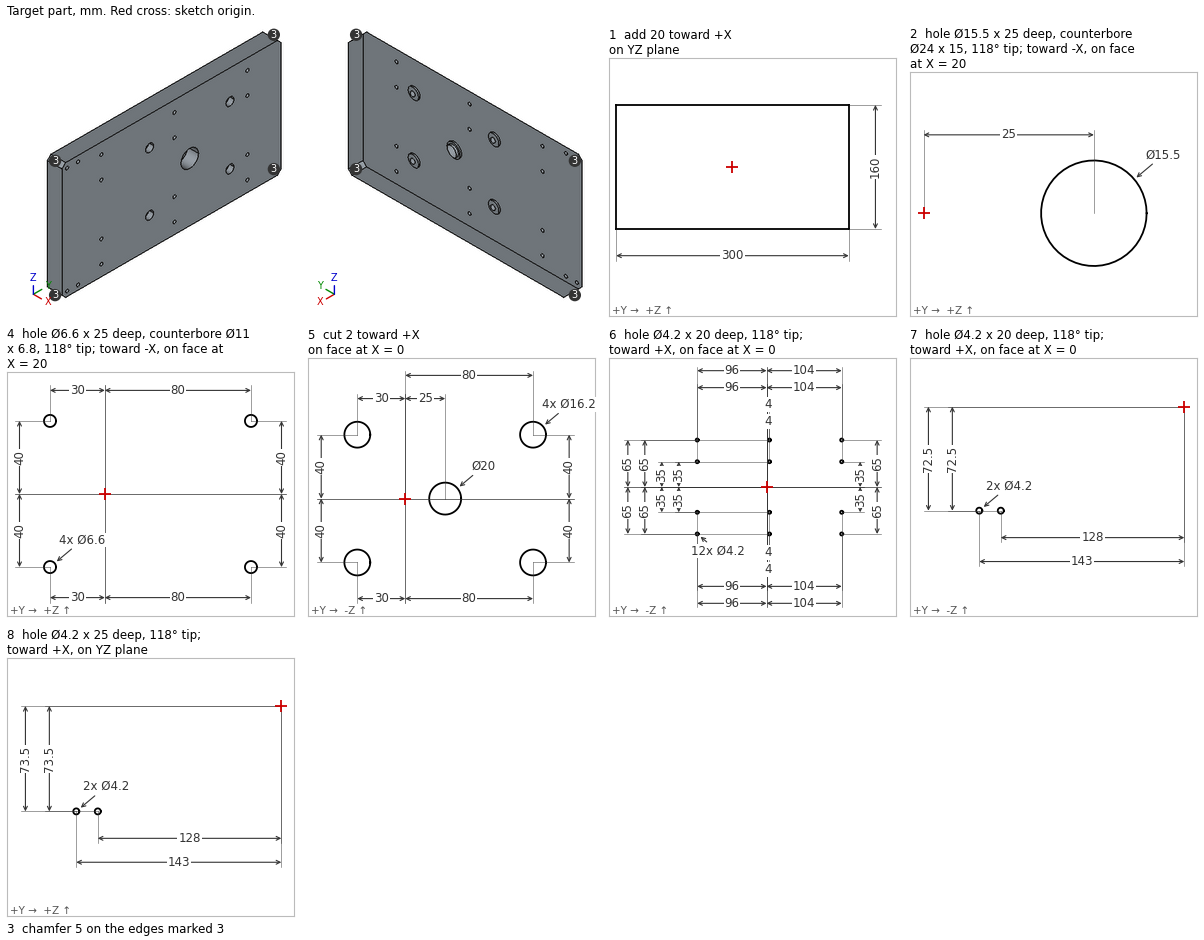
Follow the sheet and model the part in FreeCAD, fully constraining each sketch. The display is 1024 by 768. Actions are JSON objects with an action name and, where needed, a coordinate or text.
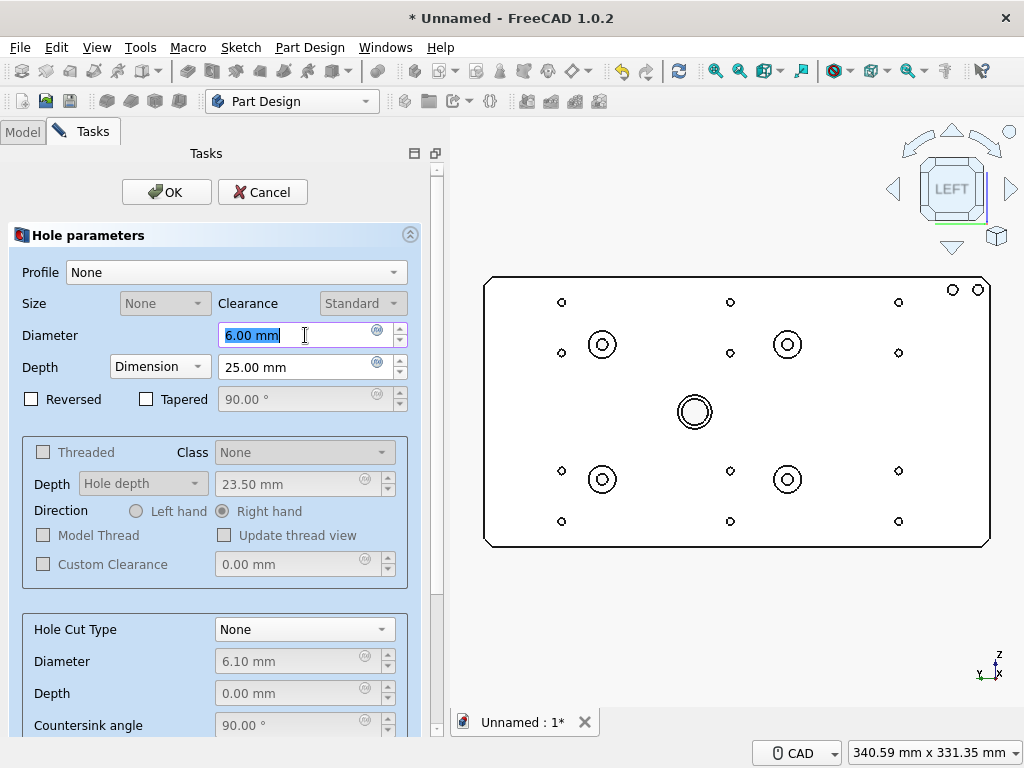
{"action": "type", "text": "4.2"}
{"action": "key", "text": "Tab"}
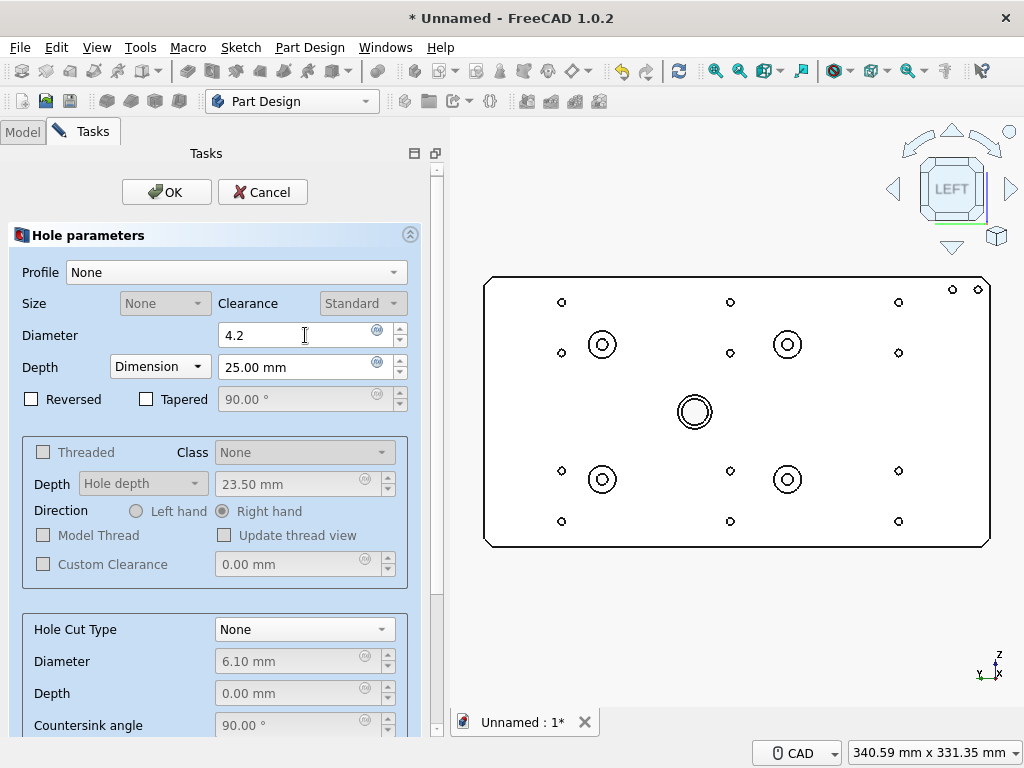
{"action": "triple_click", "coordinate": [305, 367]}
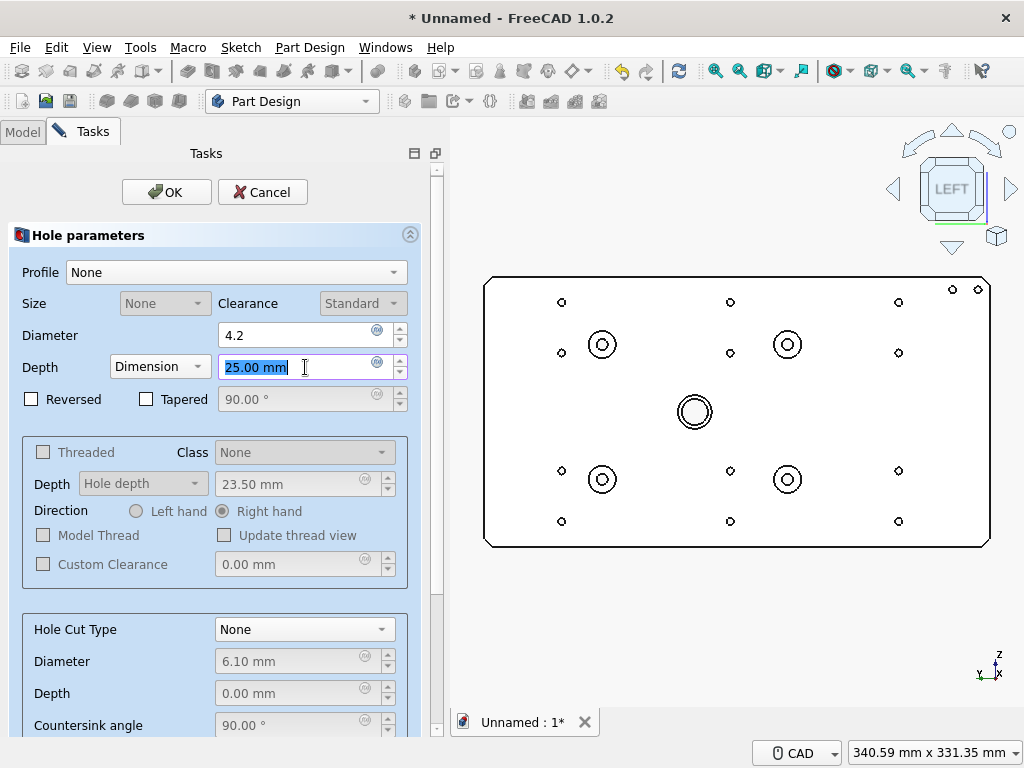
{"action": "type", "text": "20"}
{"action": "key", "text": "Tab"}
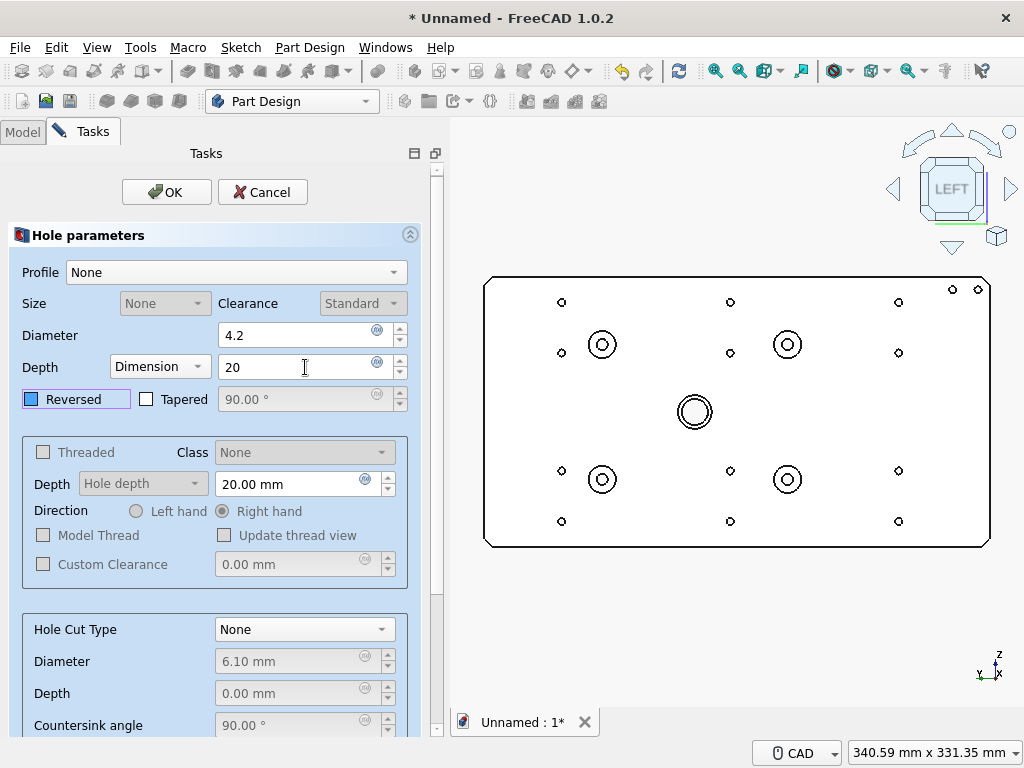
{"action": "left_click", "coordinate": [167, 192]}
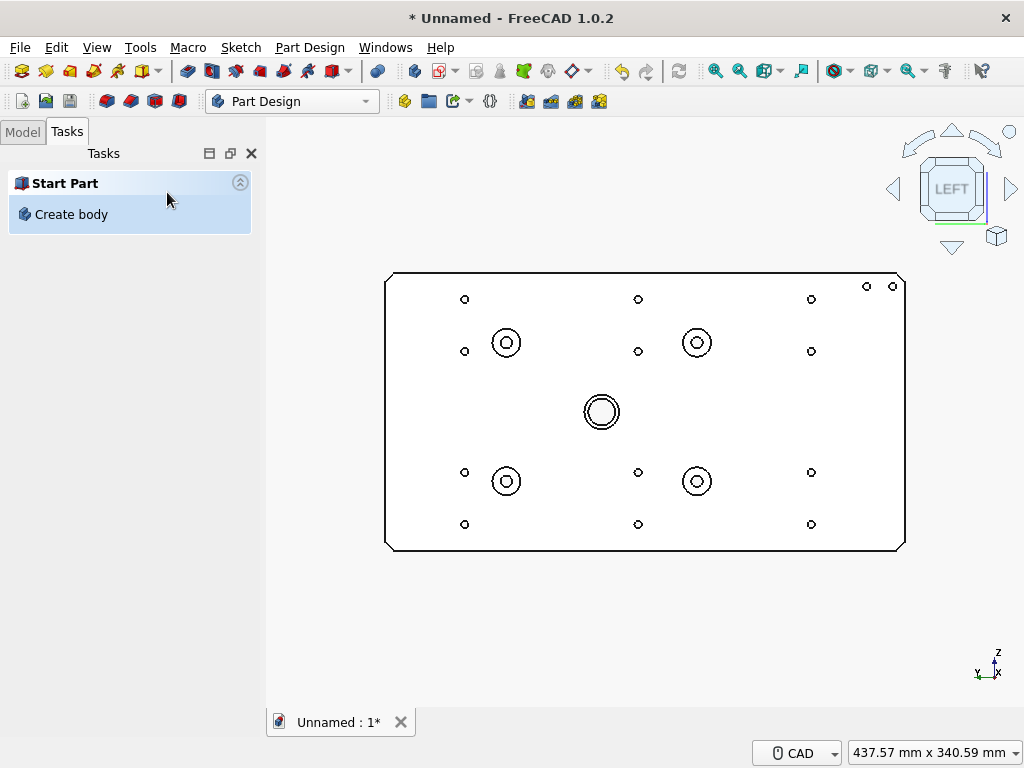
{"action": "left_click", "coordinate": [440, 72]}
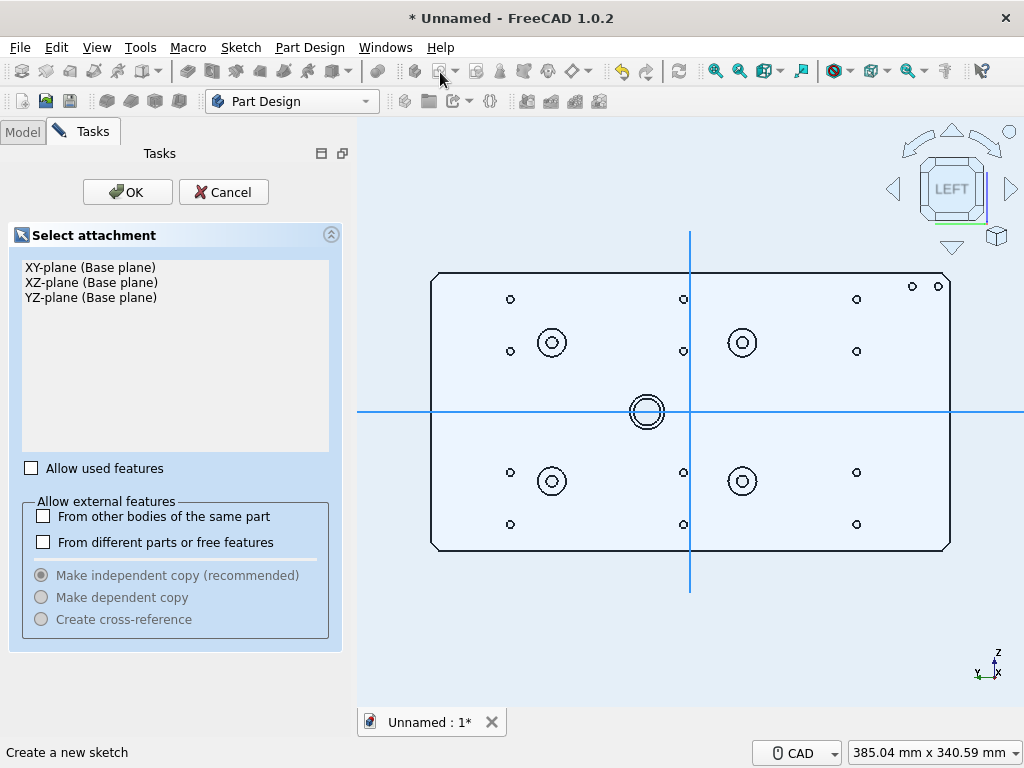
{"action": "left_click", "coordinate": [82, 298]}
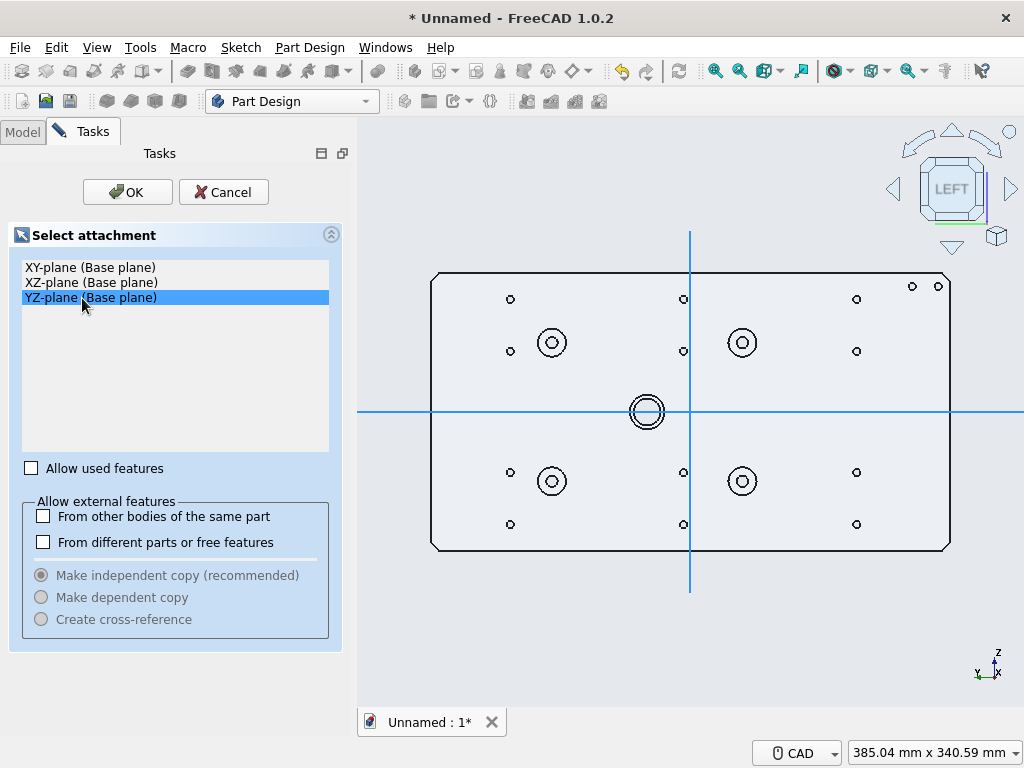
{"action": "left_click", "coordinate": [128, 192]}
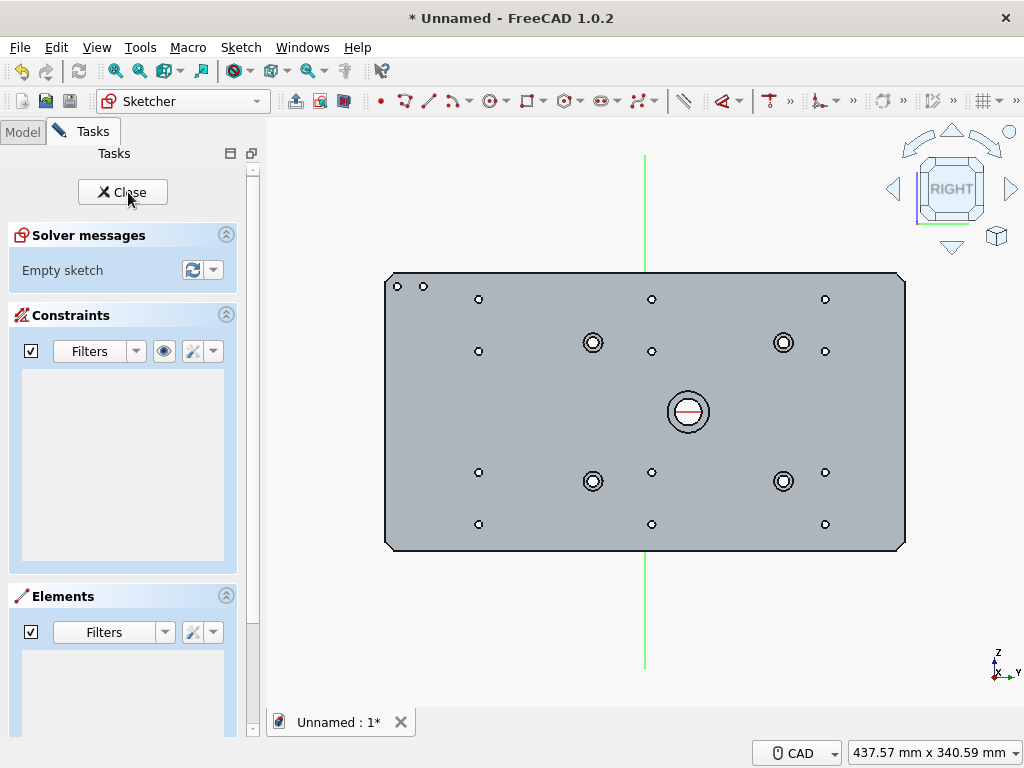
{"action": "key", "text": "q s"}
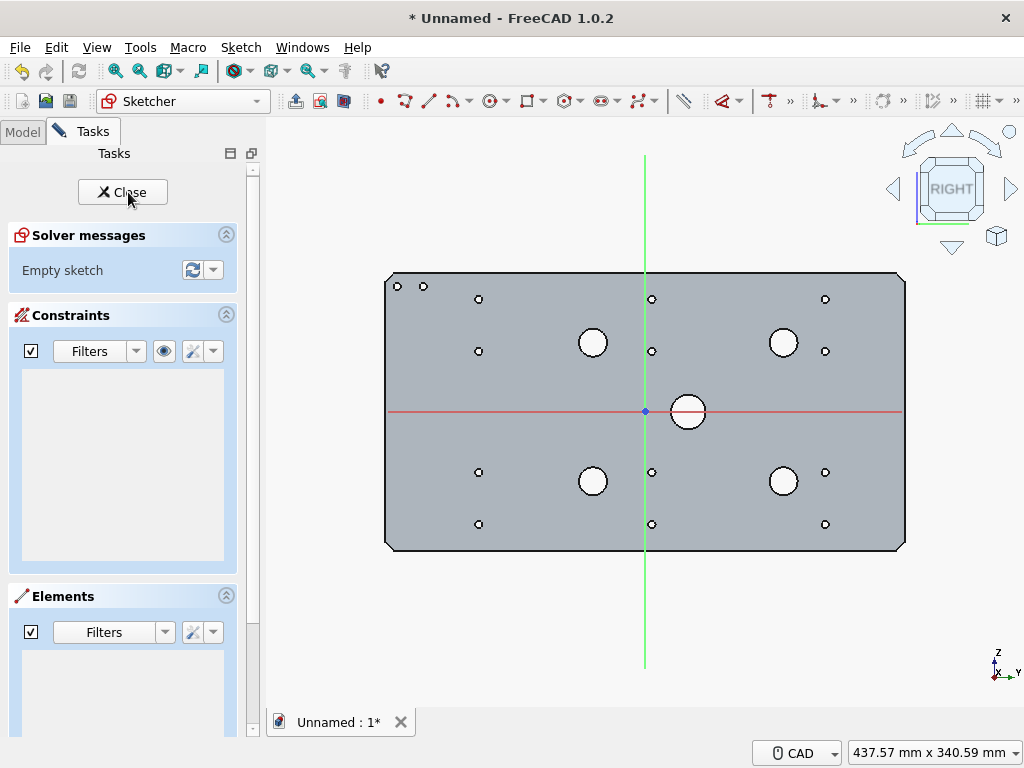
{"action": "scroll", "coordinate": [394, 552], "scroll_direction": "up", "scroll_amount": 12}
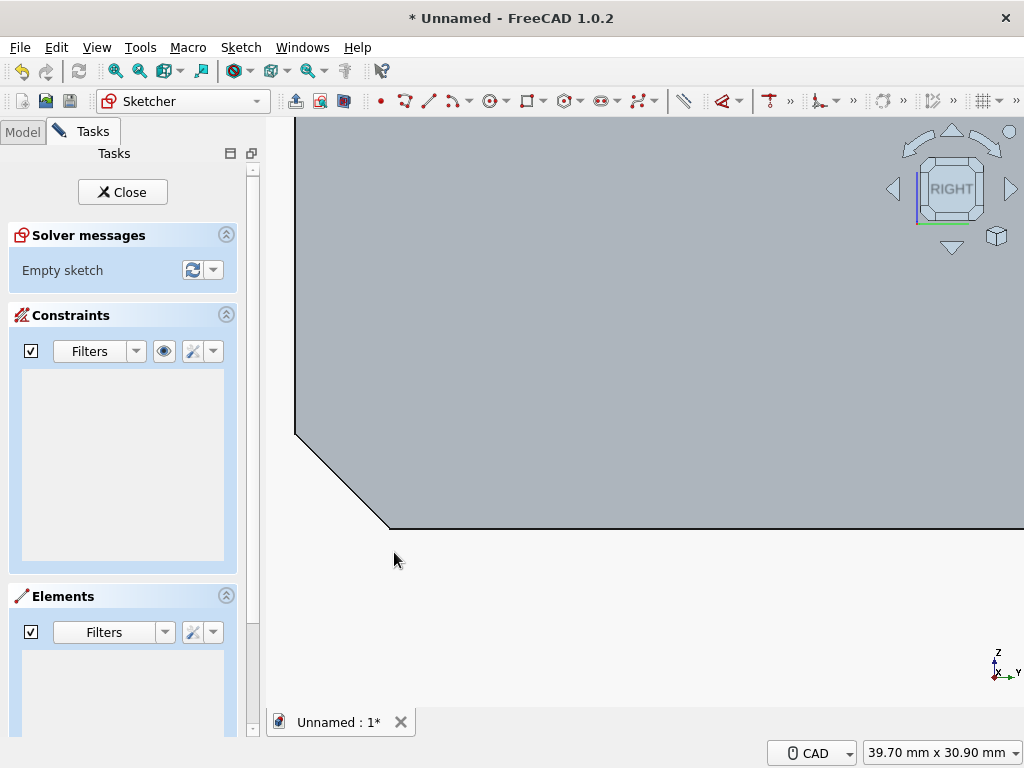
{"action": "key", "text": "g c"}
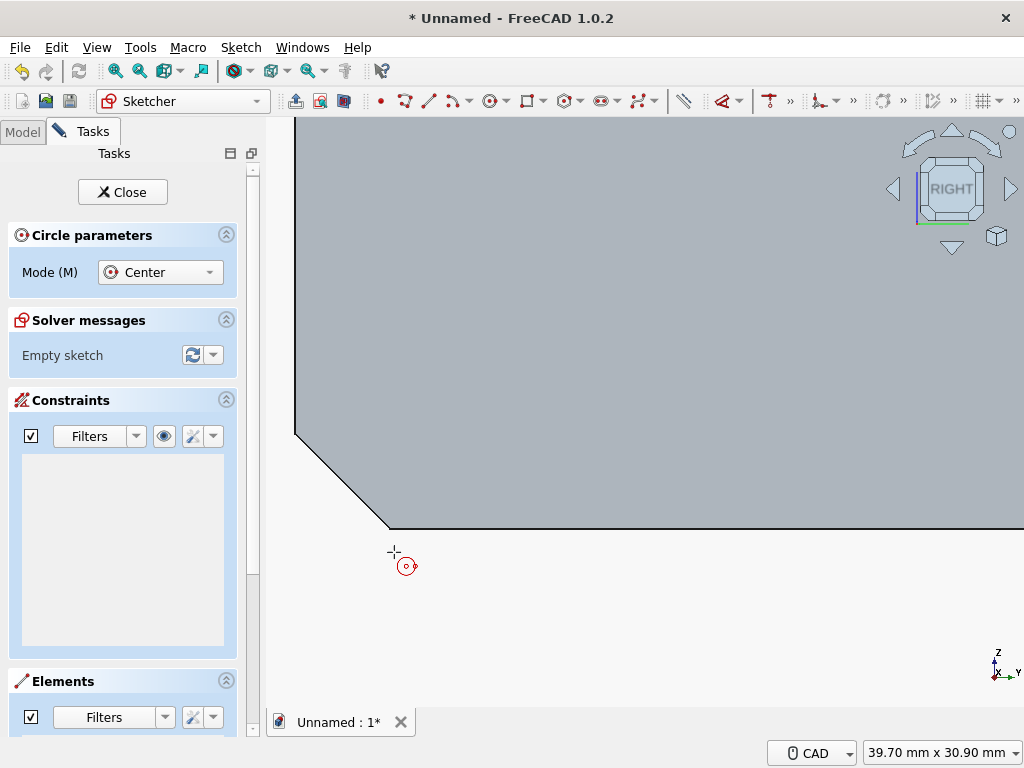
{"action": "left_click", "coordinate": [428, 405]}
{"action": "left_click", "coordinate": [457, 377]}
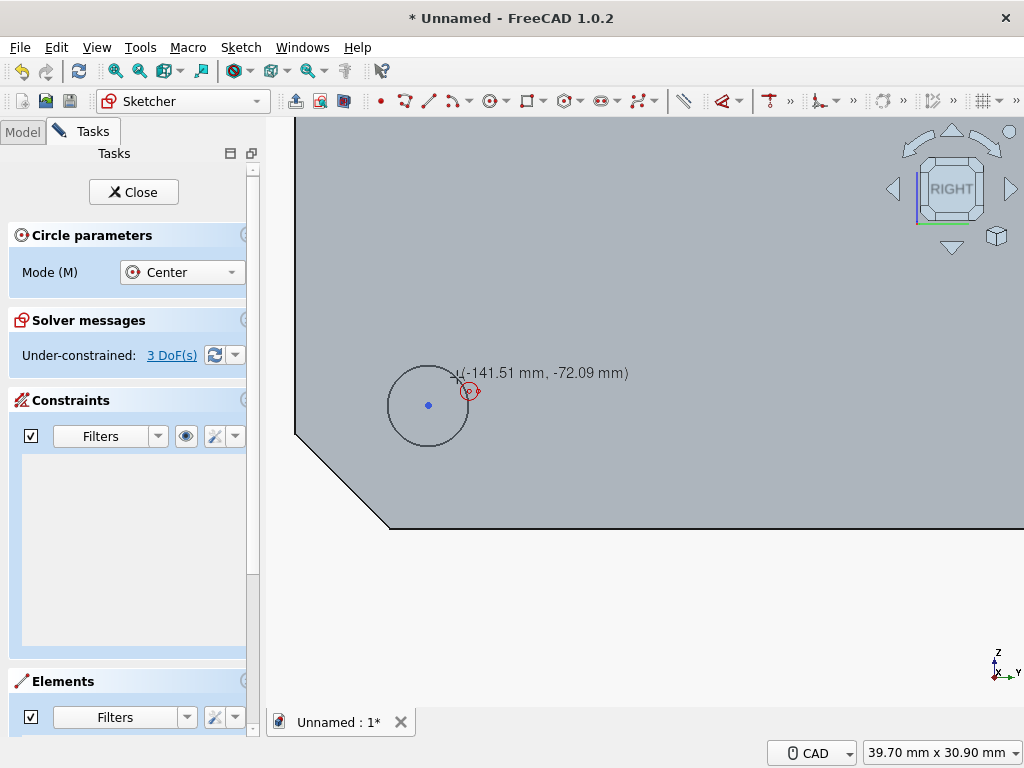
{"action": "left_click", "coordinate": [715, 405]}
{"action": "left_click", "coordinate": [743, 377]}
{"action": "key", "text": "Escape"}